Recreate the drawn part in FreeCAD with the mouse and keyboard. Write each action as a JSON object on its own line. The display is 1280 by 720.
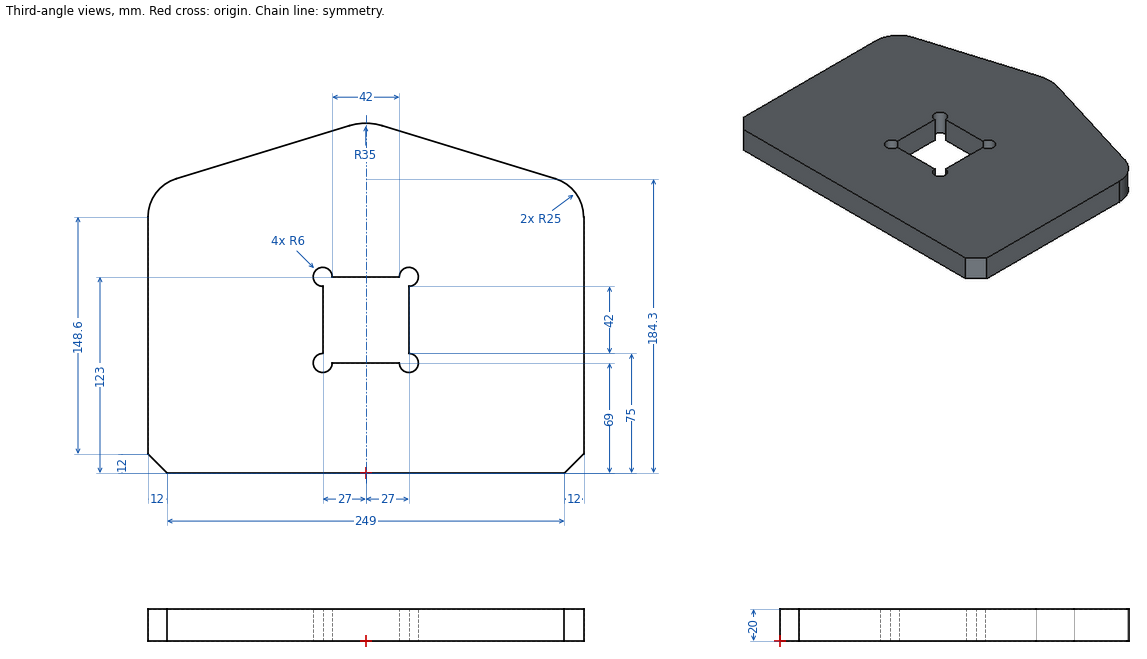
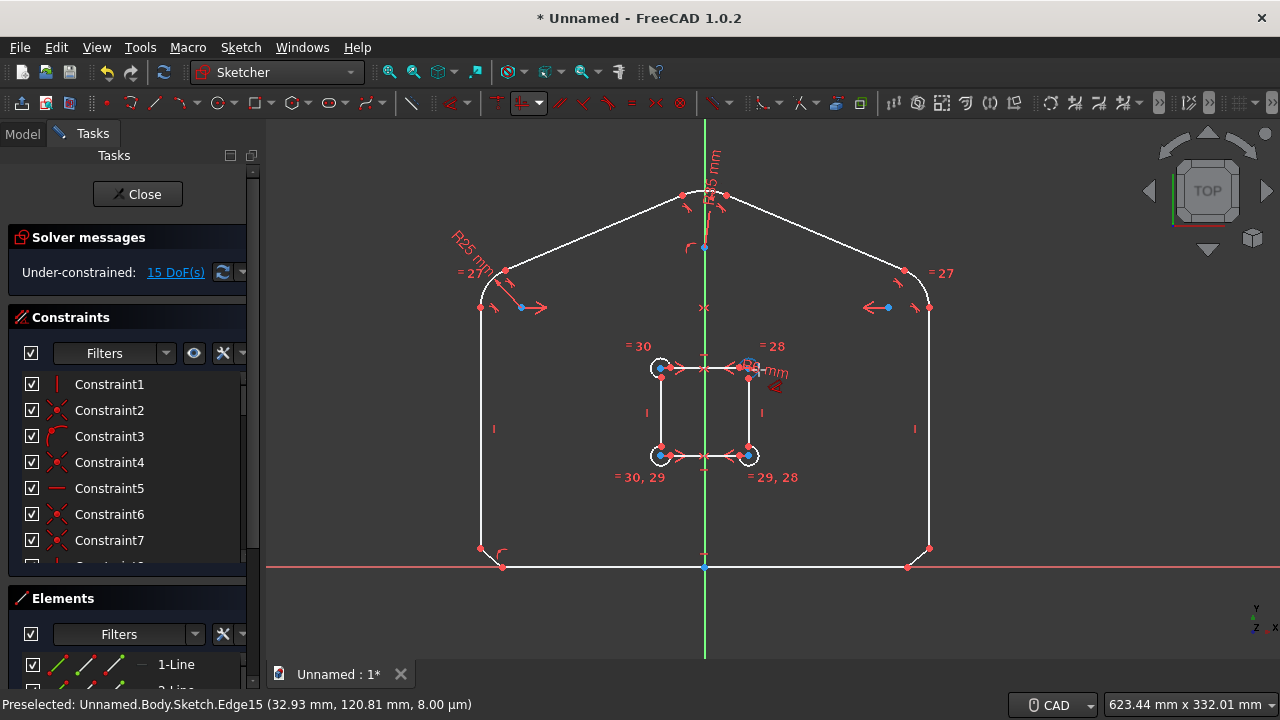
{"action": "left_click", "coordinate": [691, 368]}
{"action": "left_click", "coordinate": [689, 334]}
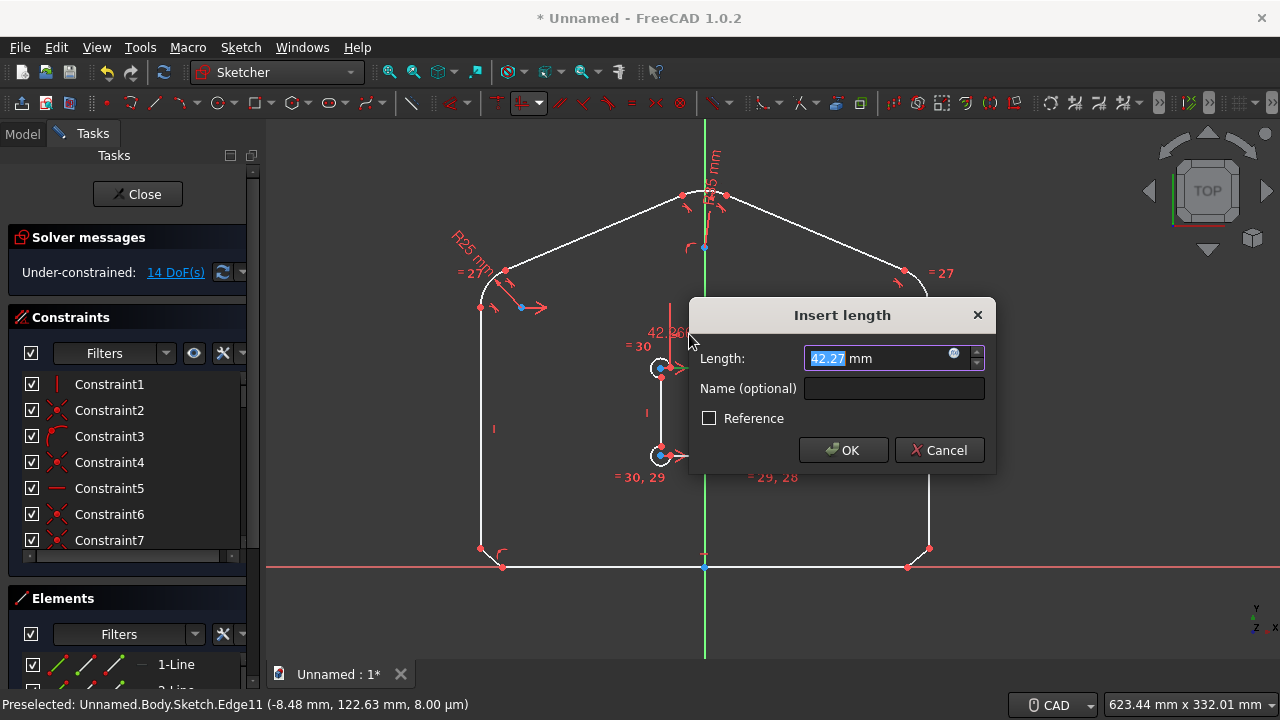
{"action": "type", "text": "42"}
{"action": "key", "text": "Return"}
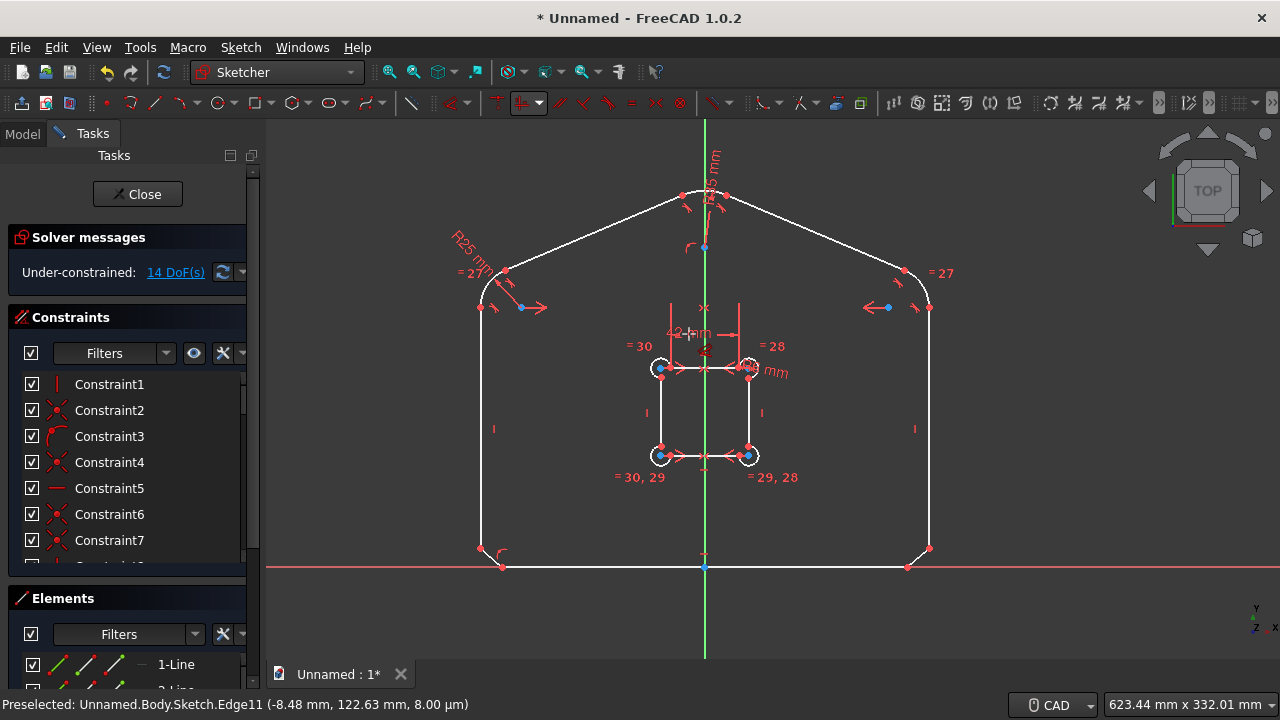
{"action": "left_click", "coordinate": [749, 398]}
{"action": "left_click", "coordinate": [783, 412]}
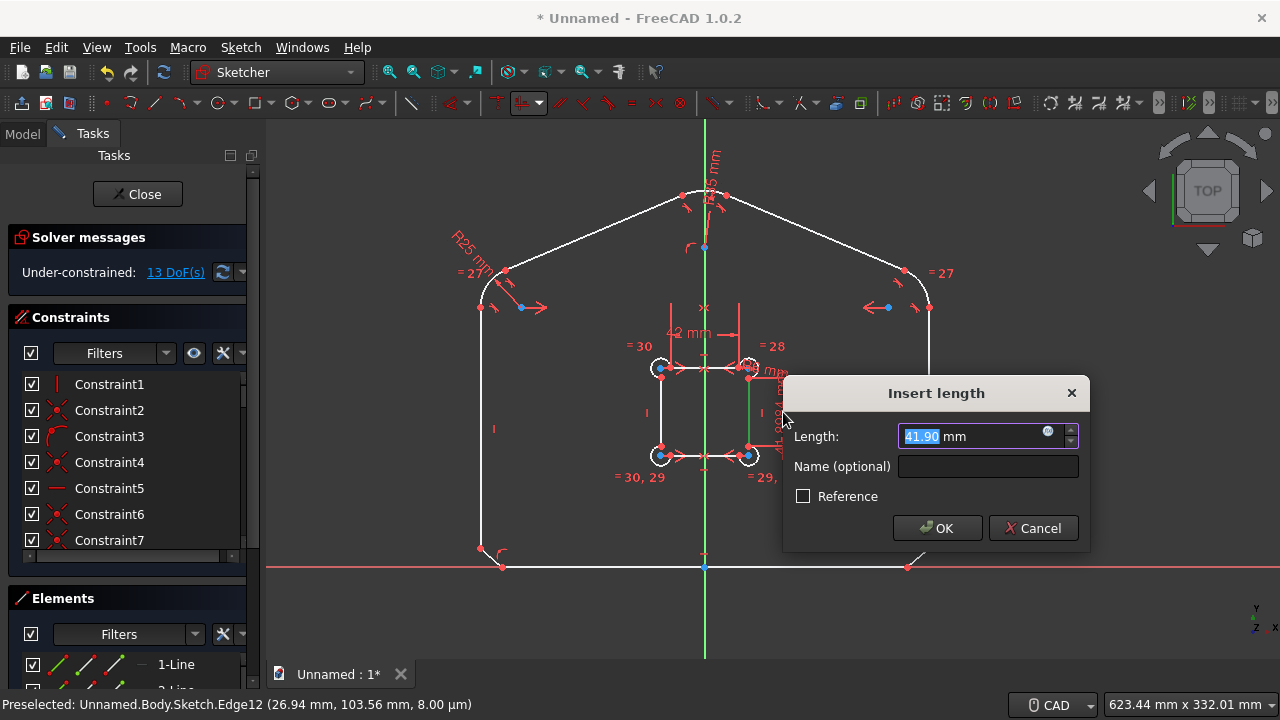
{"action": "type", "text": "42"}
{"action": "key", "text": "Return"}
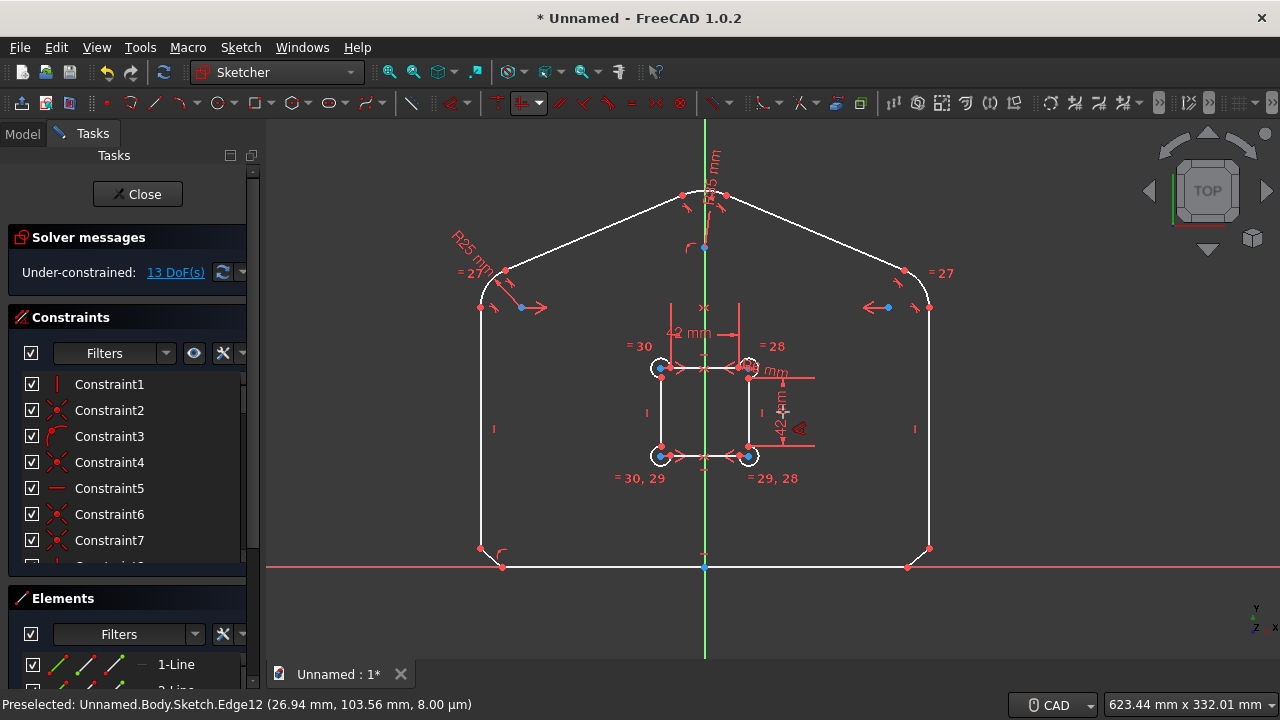
{"action": "left_click", "coordinate": [718, 456]}
{"action": "left_click", "coordinate": [689, 490]}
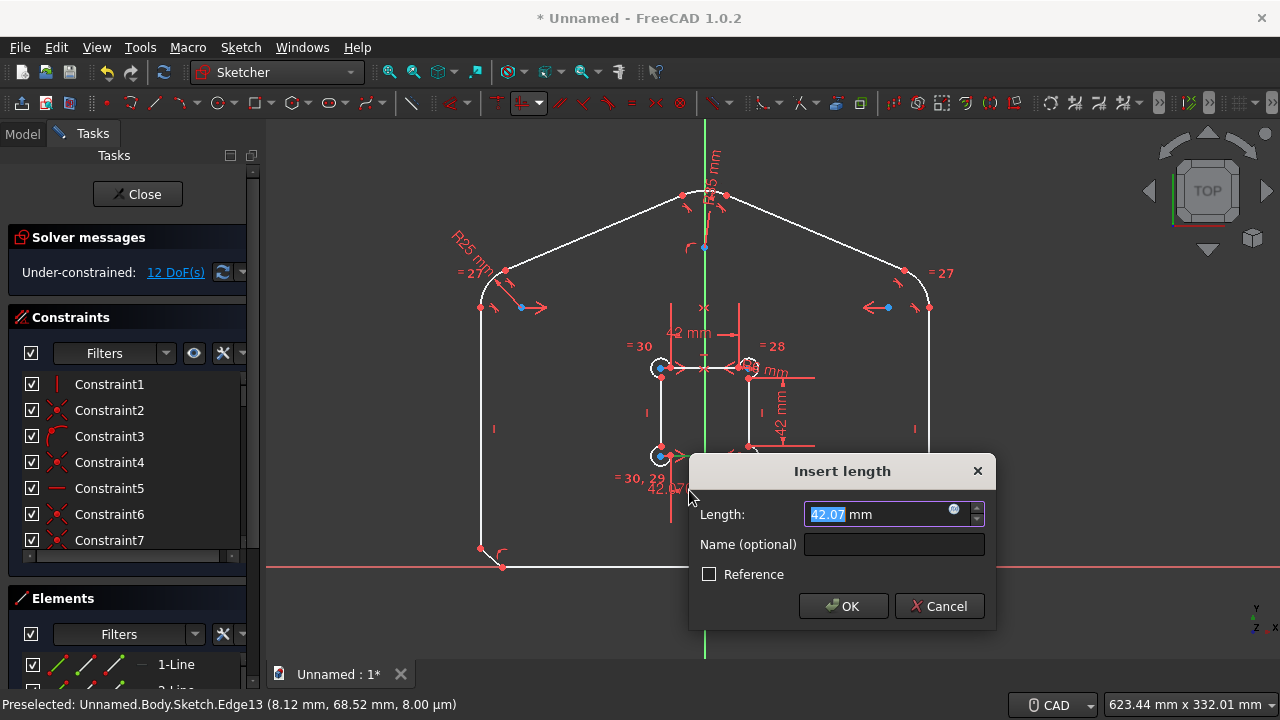
{"action": "type", "text": "42"}
{"action": "key", "text": "Return"}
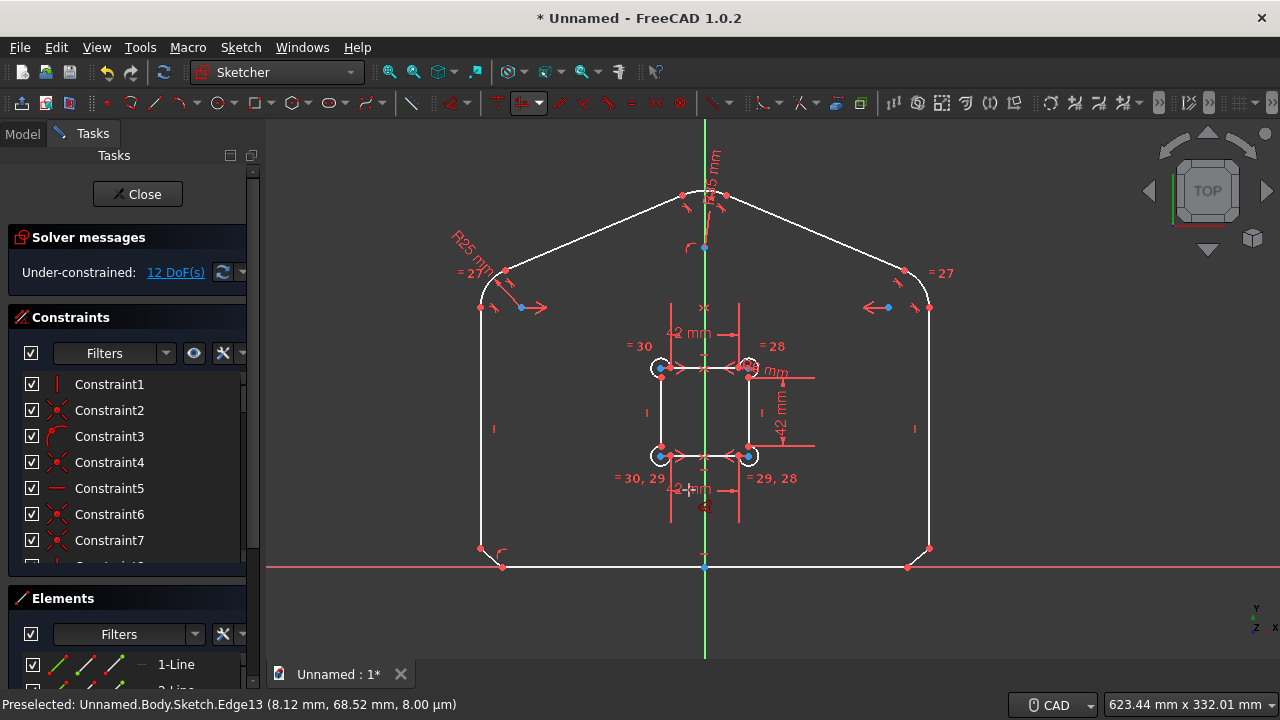
{"action": "left_click", "coordinate": [624, 567]}
{"action": "left_click", "coordinate": [611, 601]}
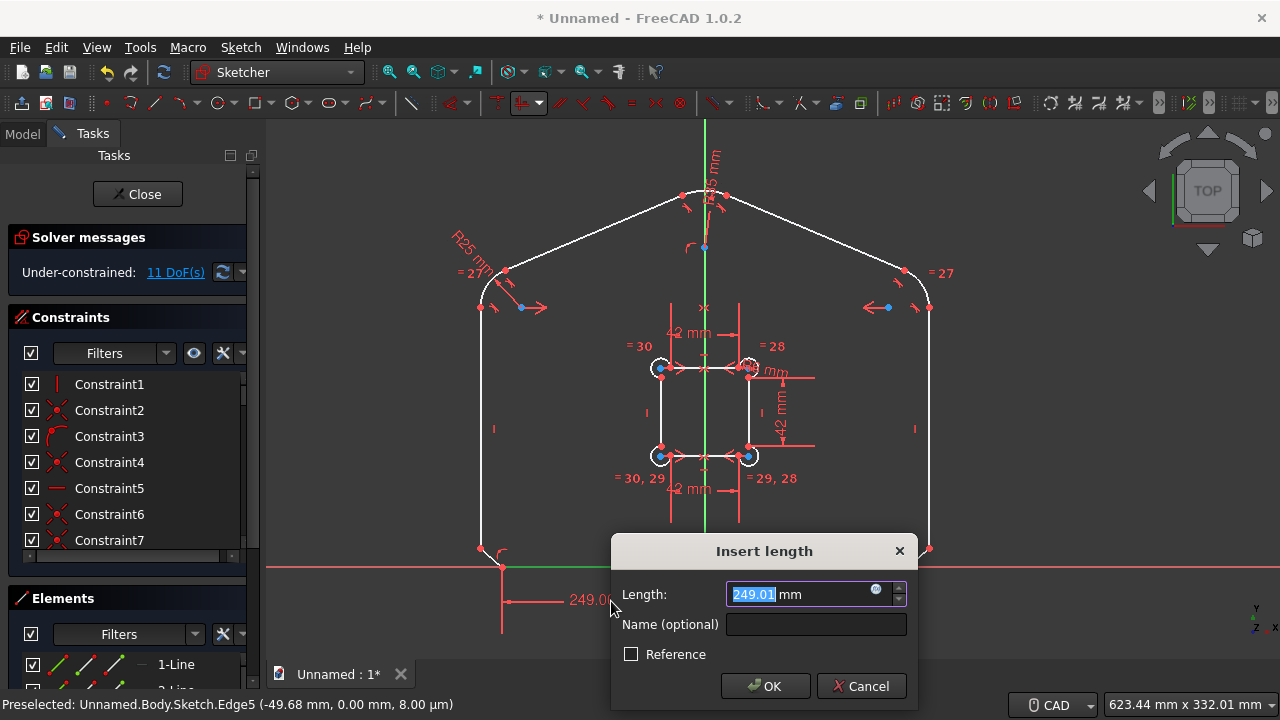
{"action": "type", "text": "249"}
{"action": "key", "text": "Return"}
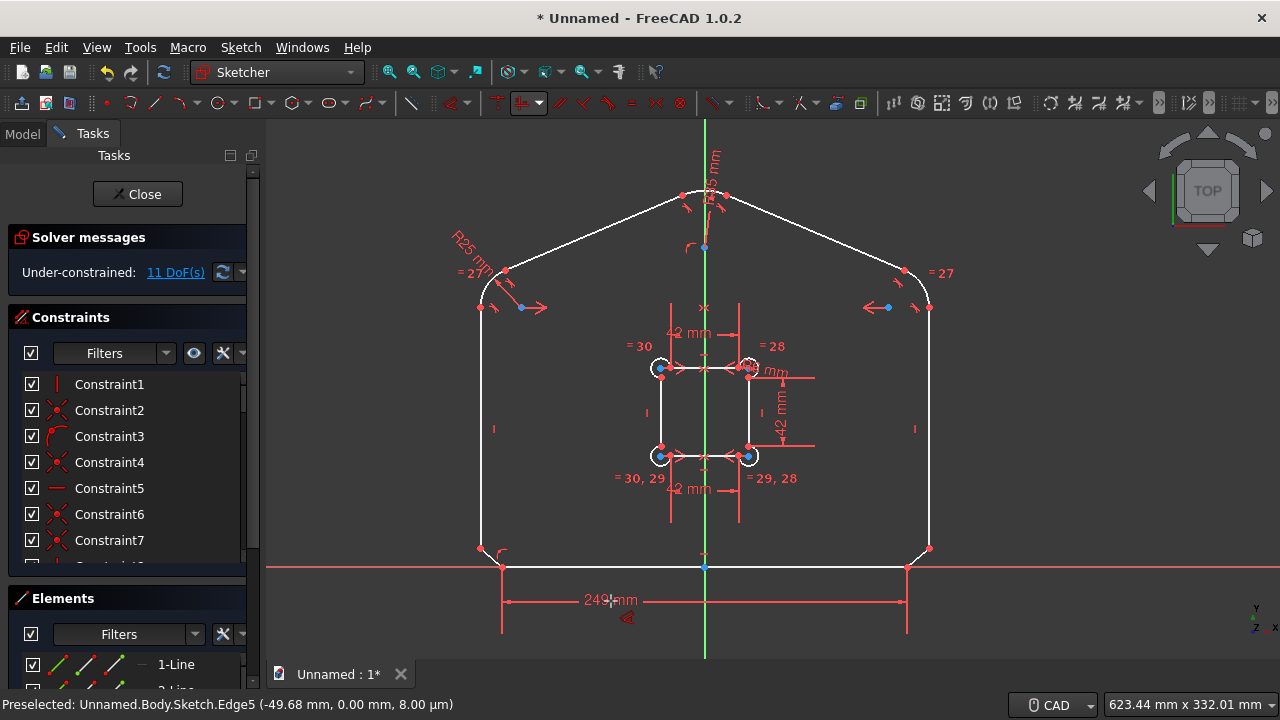
{"action": "scroll", "coordinate": [481, 549], "scroll_direction": "up", "scroll_amount": 4}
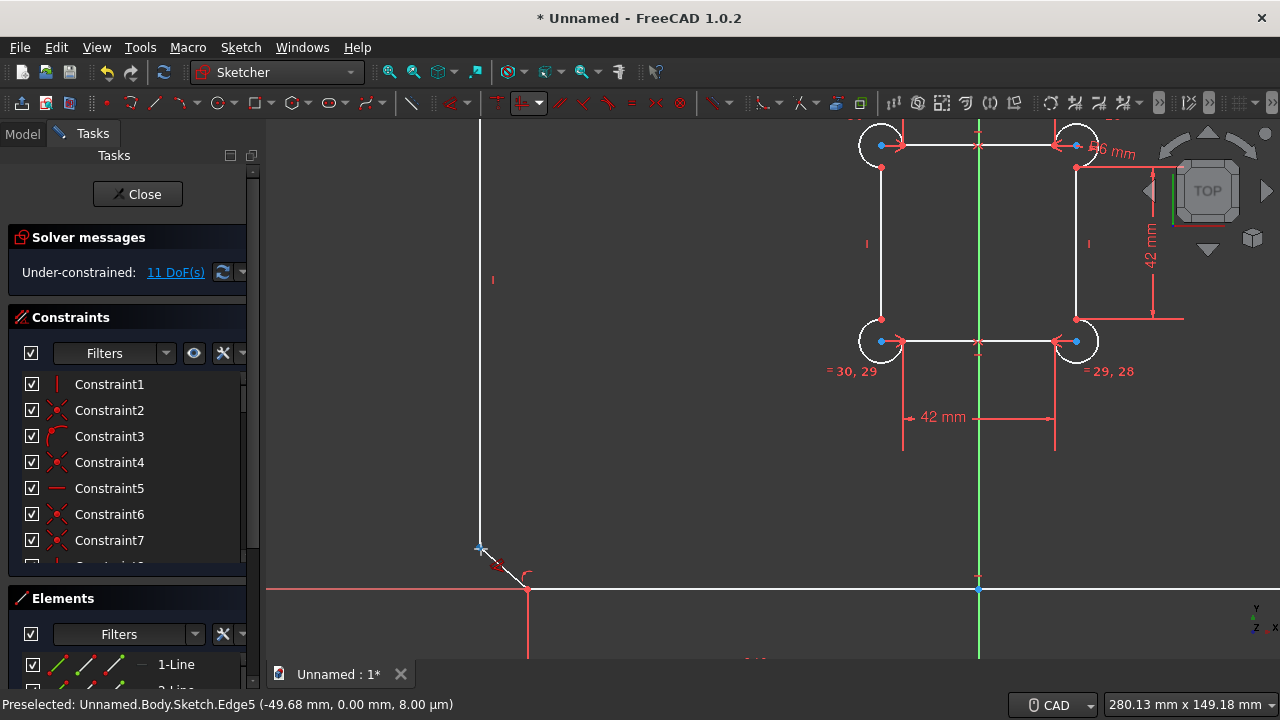
{"action": "left_click", "coordinate": [480, 547]}
{"action": "left_click", "coordinate": [446, 568]}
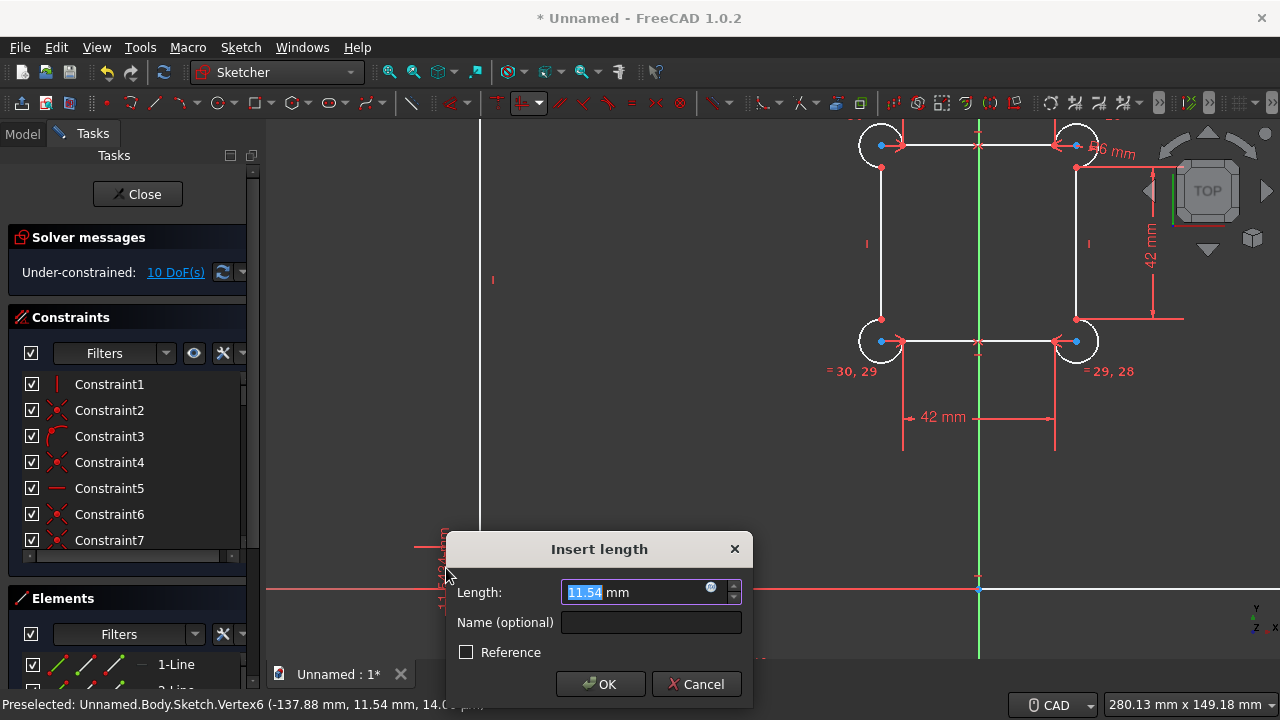
{"action": "type", "text": "12"}
{"action": "key", "text": "Return"}